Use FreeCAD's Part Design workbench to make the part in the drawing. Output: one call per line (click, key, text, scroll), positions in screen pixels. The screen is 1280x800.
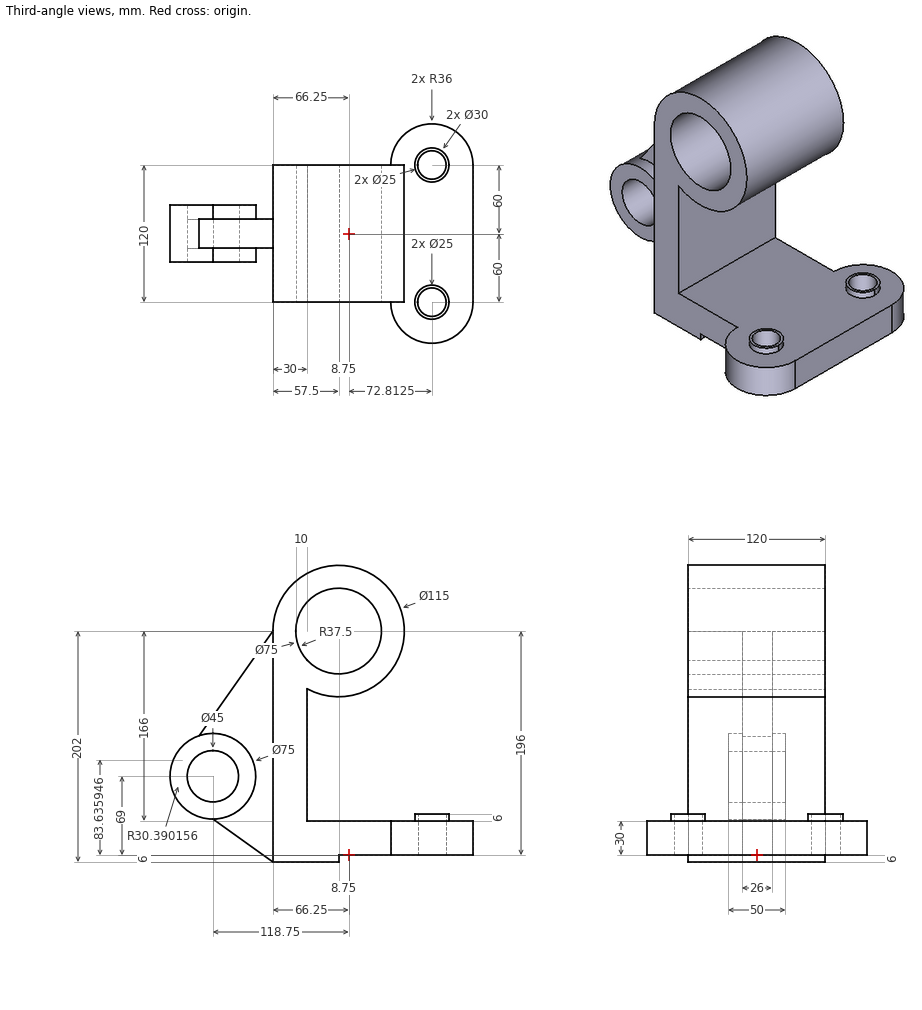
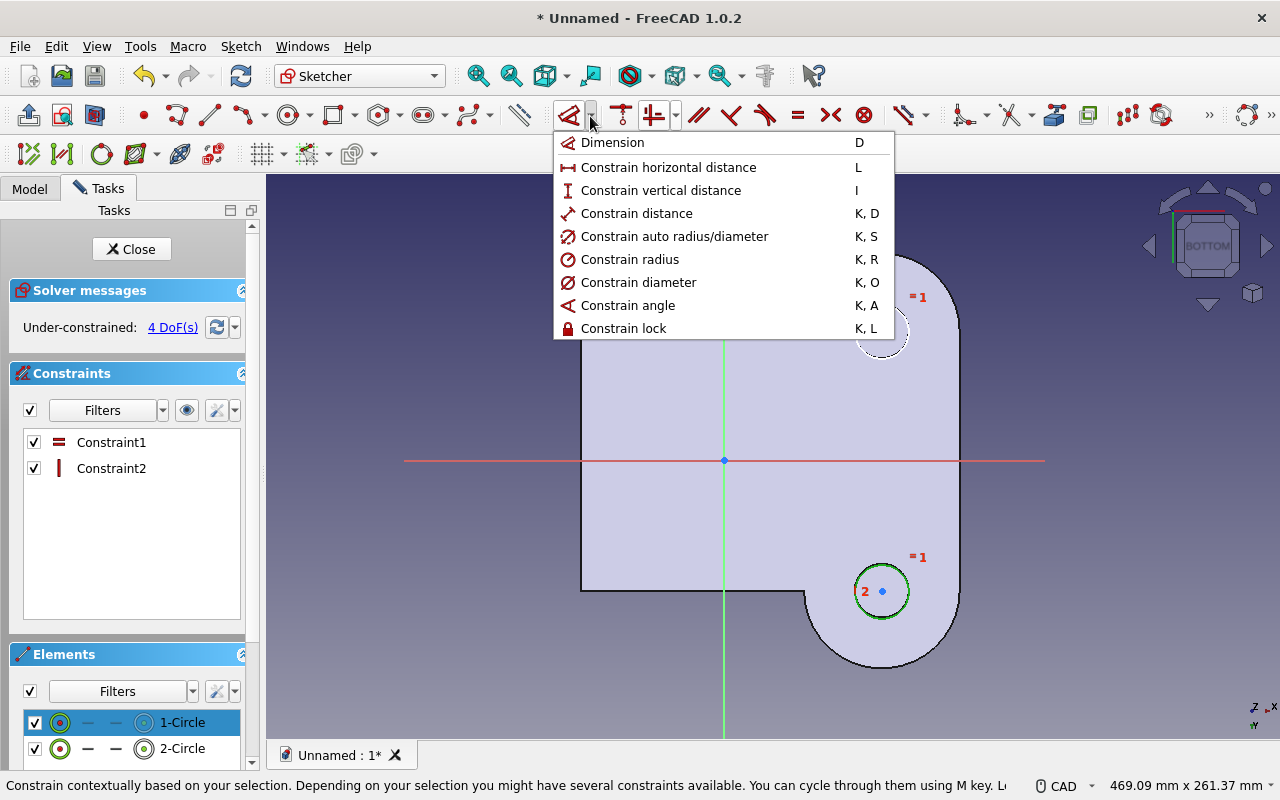
click(724, 282)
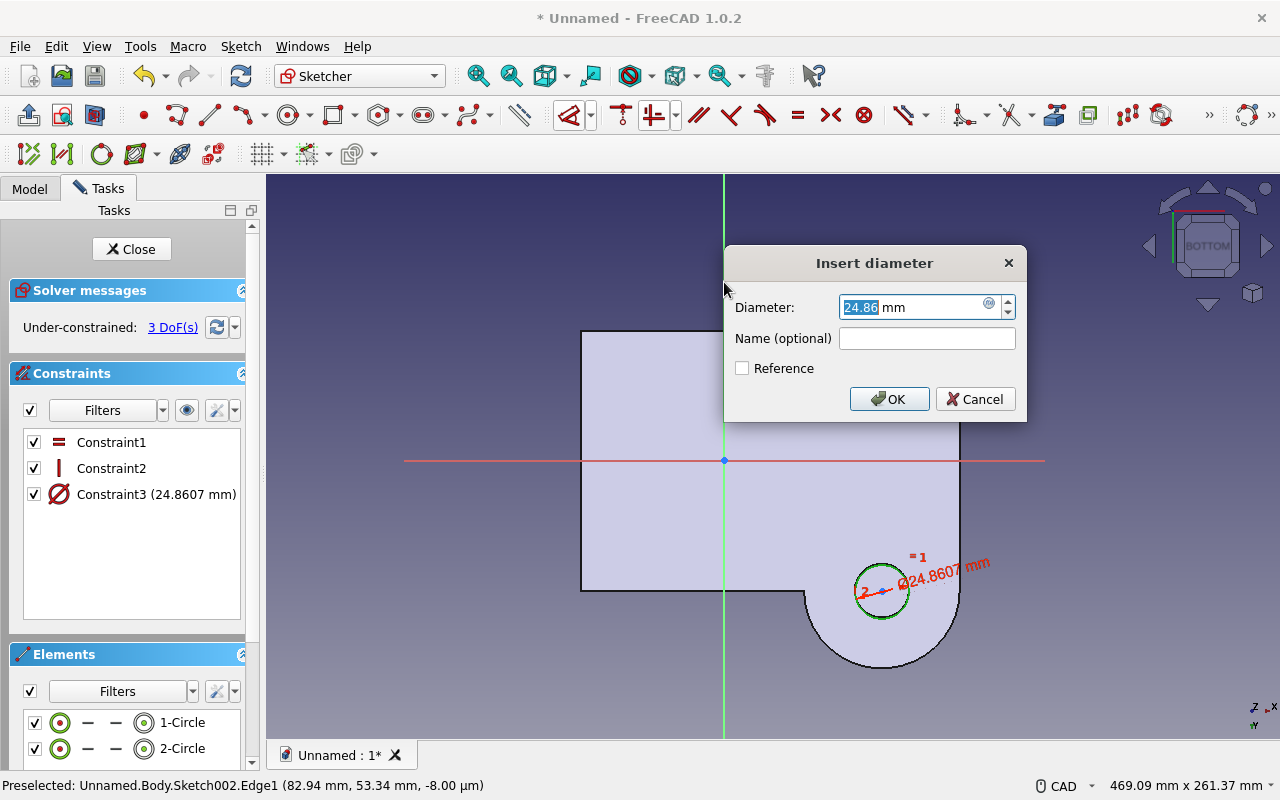
text(25)
key(Return)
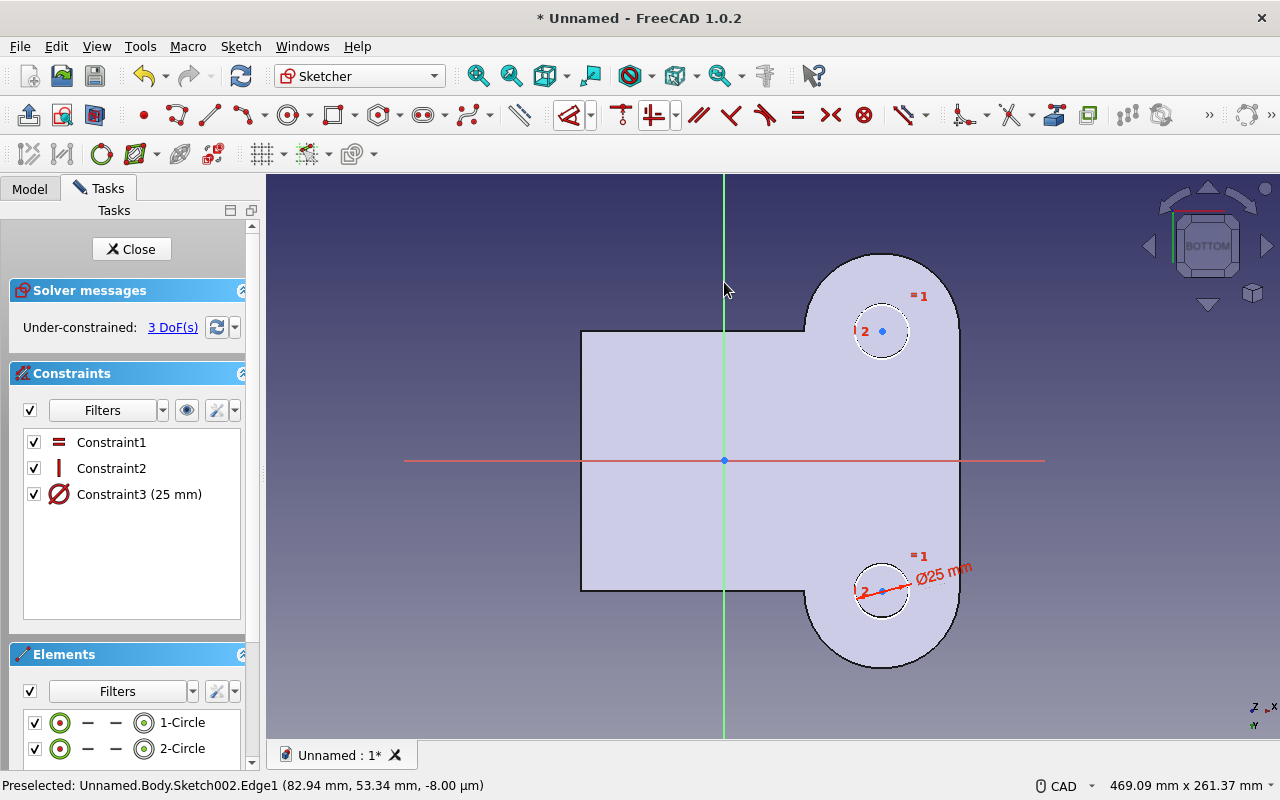
click(882, 592)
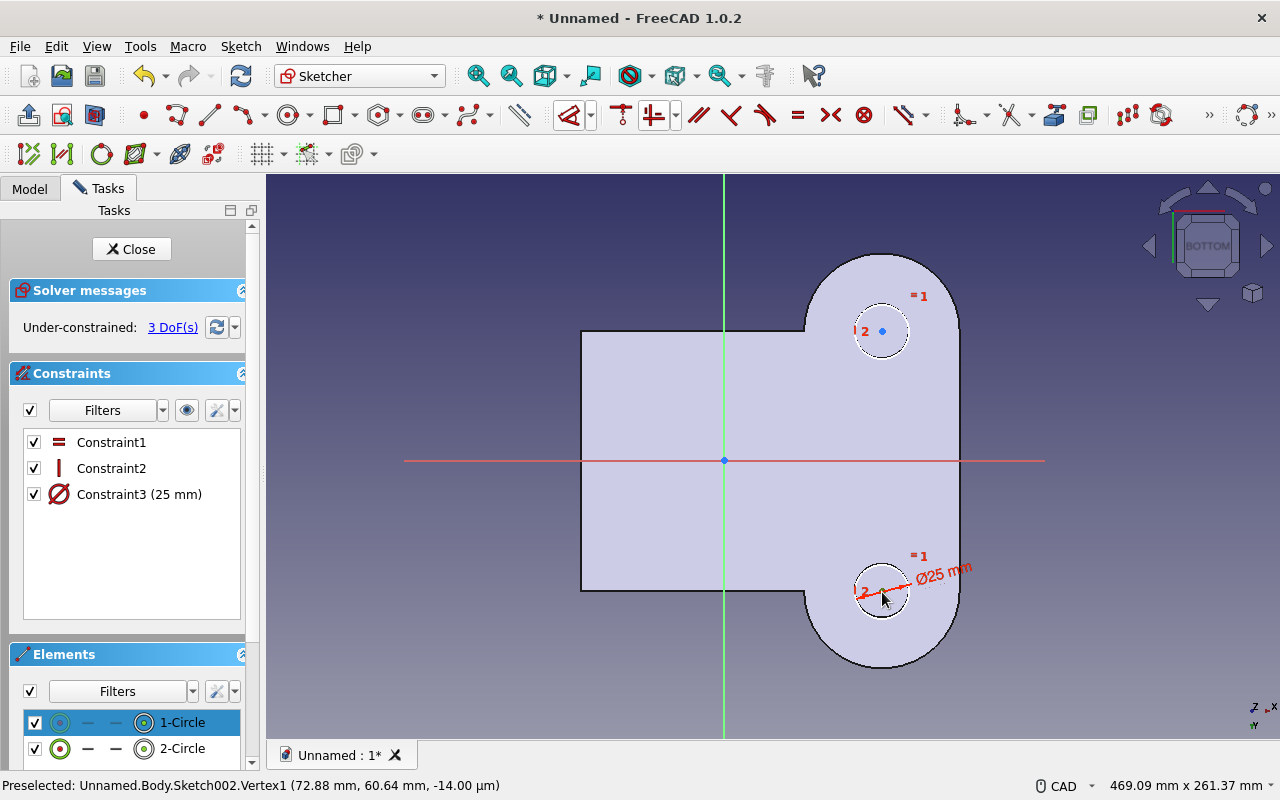
key(i)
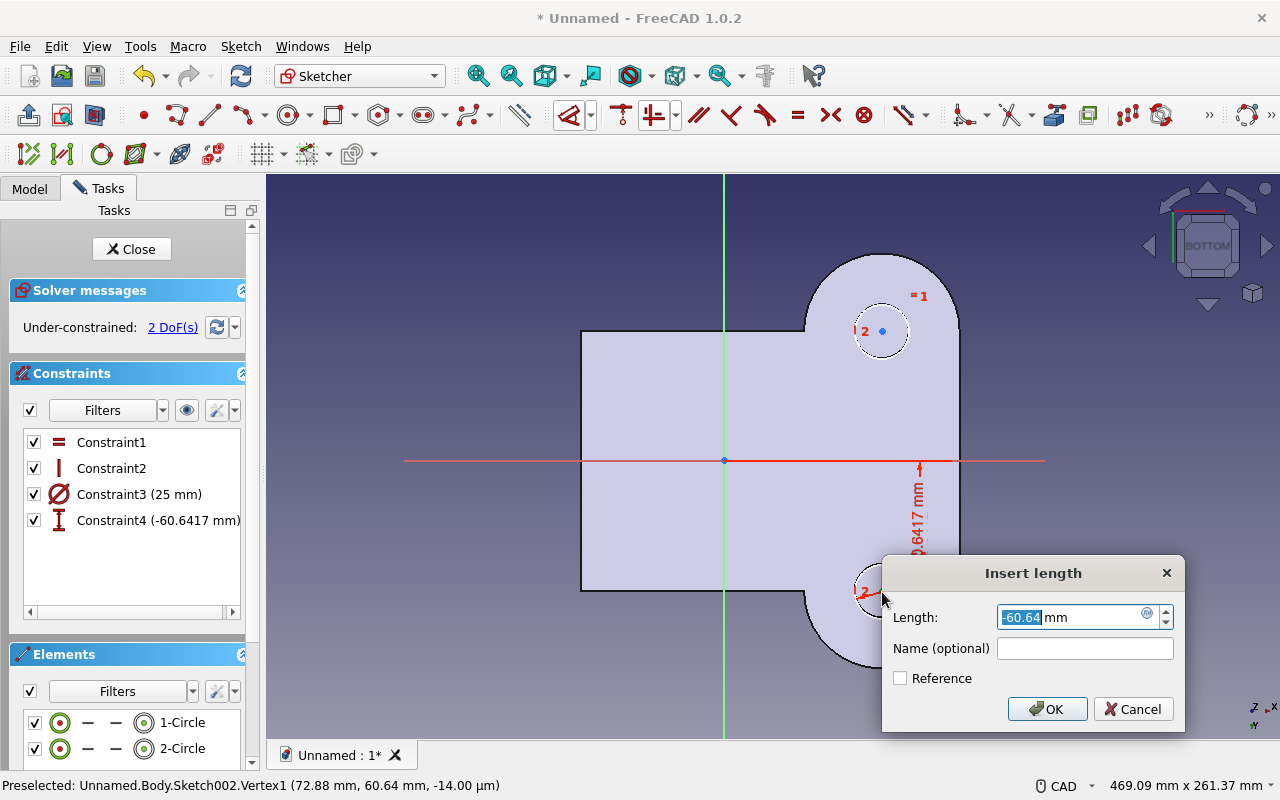
text(-60)
key(Return)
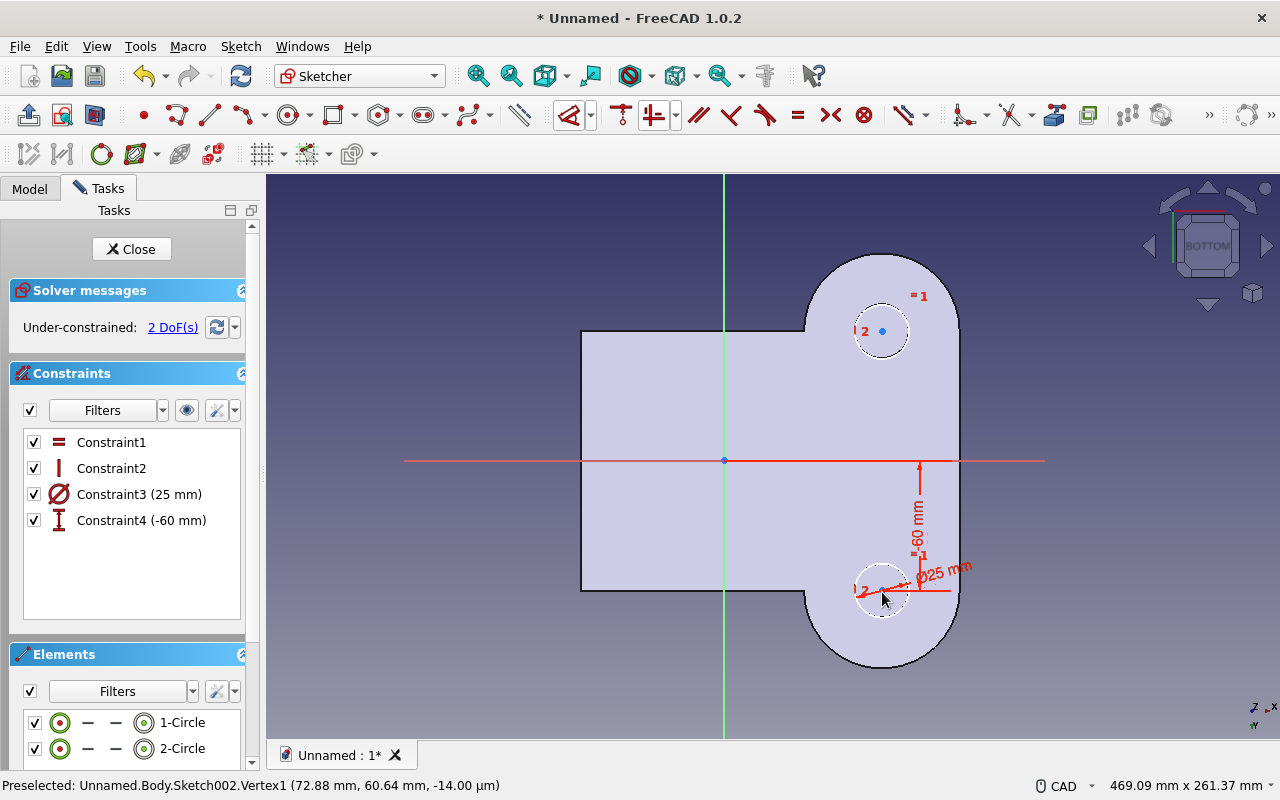
click(882, 332)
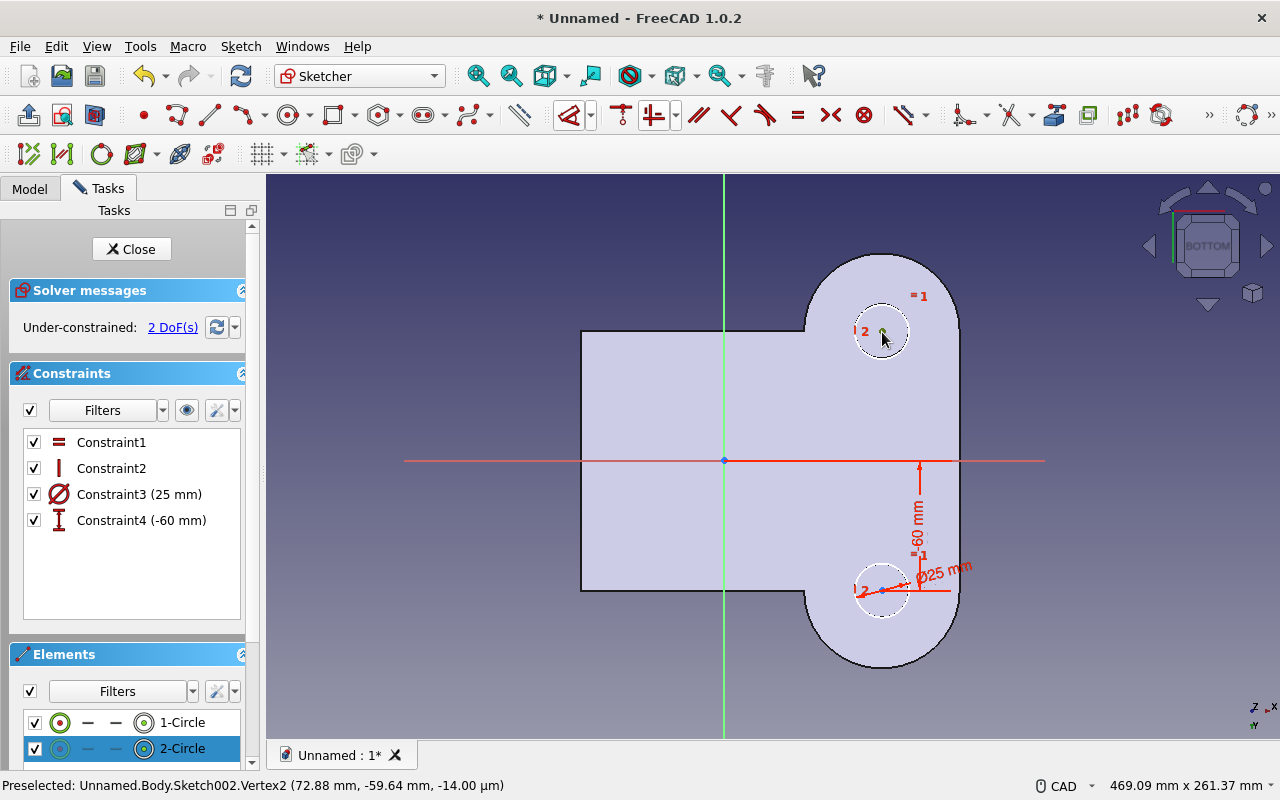
key(i)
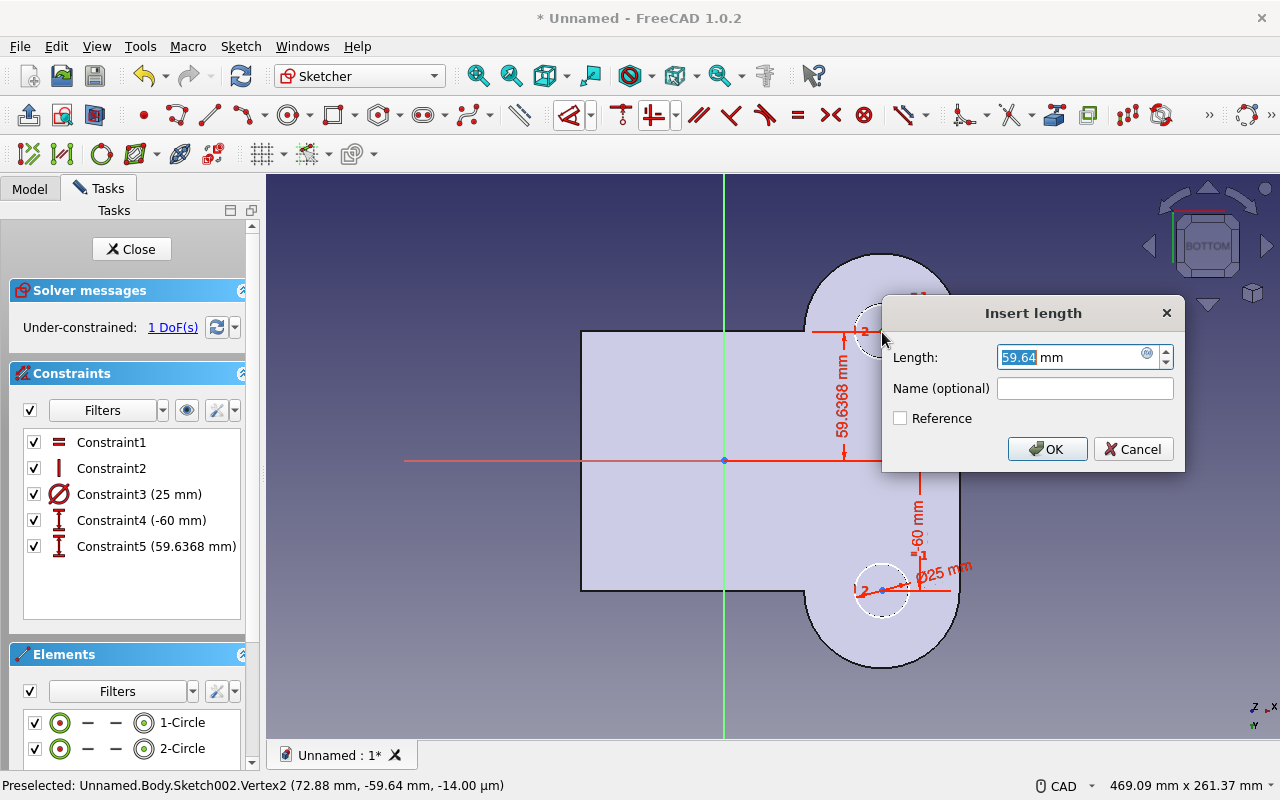
text(60)
key(Return)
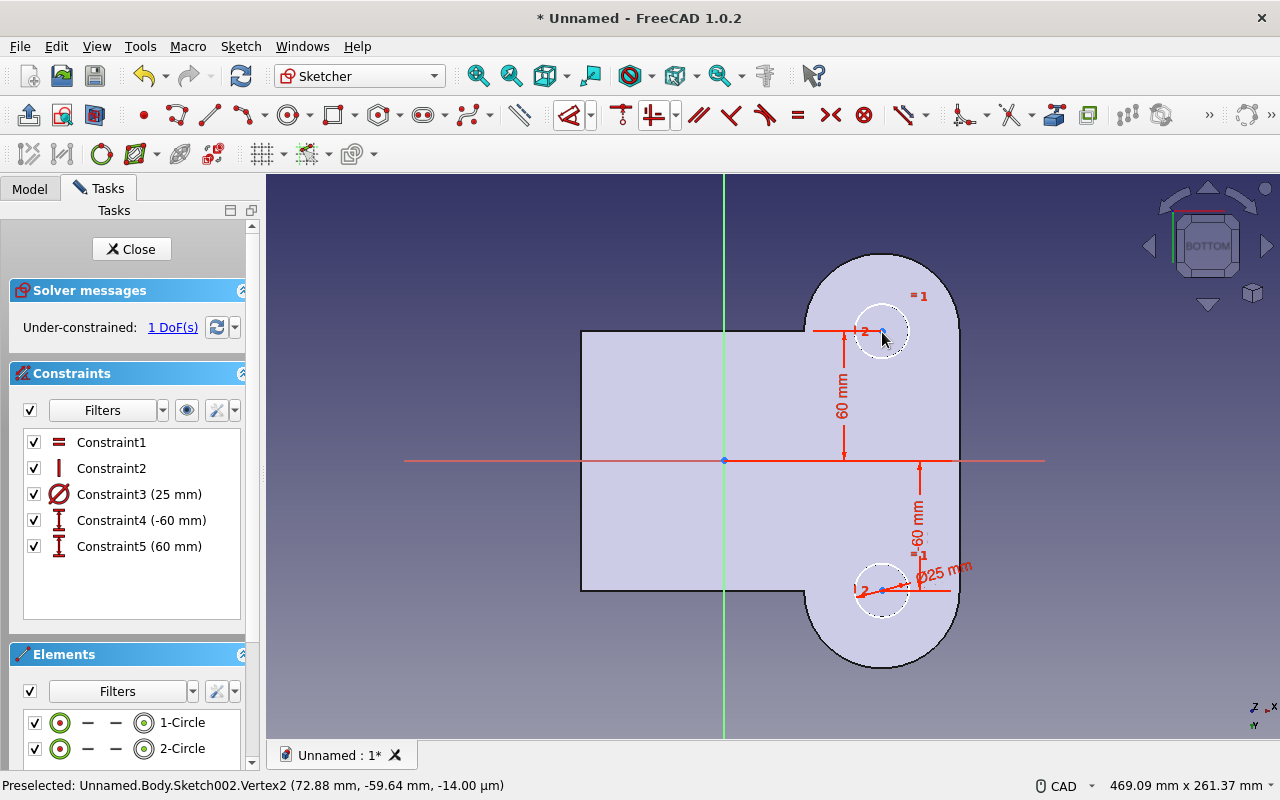
click(882, 591)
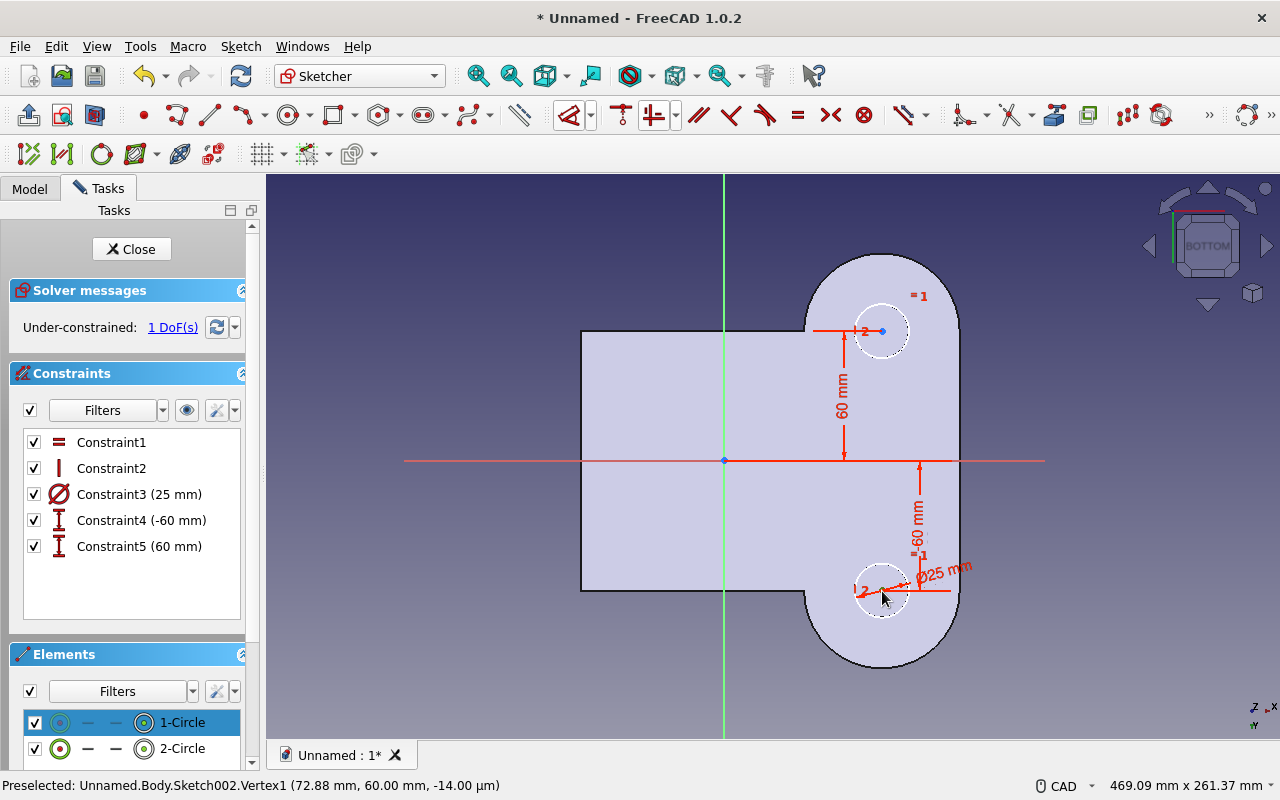
click(590, 116)